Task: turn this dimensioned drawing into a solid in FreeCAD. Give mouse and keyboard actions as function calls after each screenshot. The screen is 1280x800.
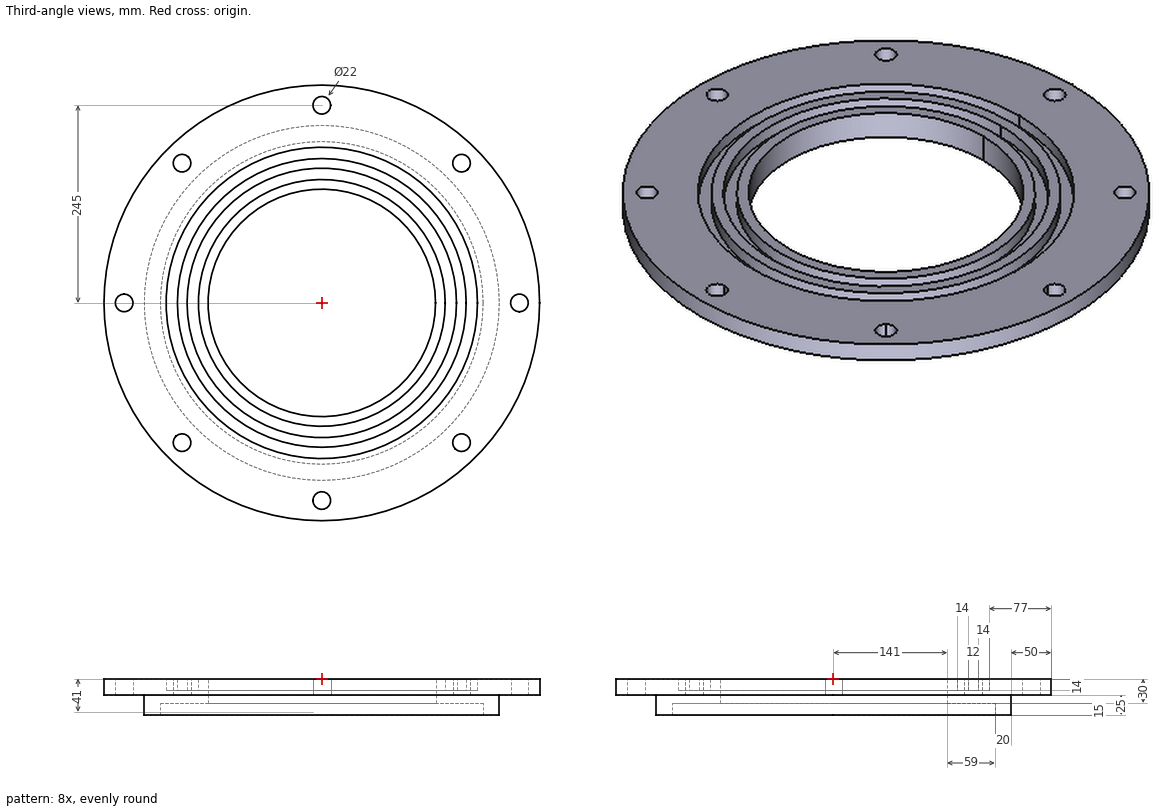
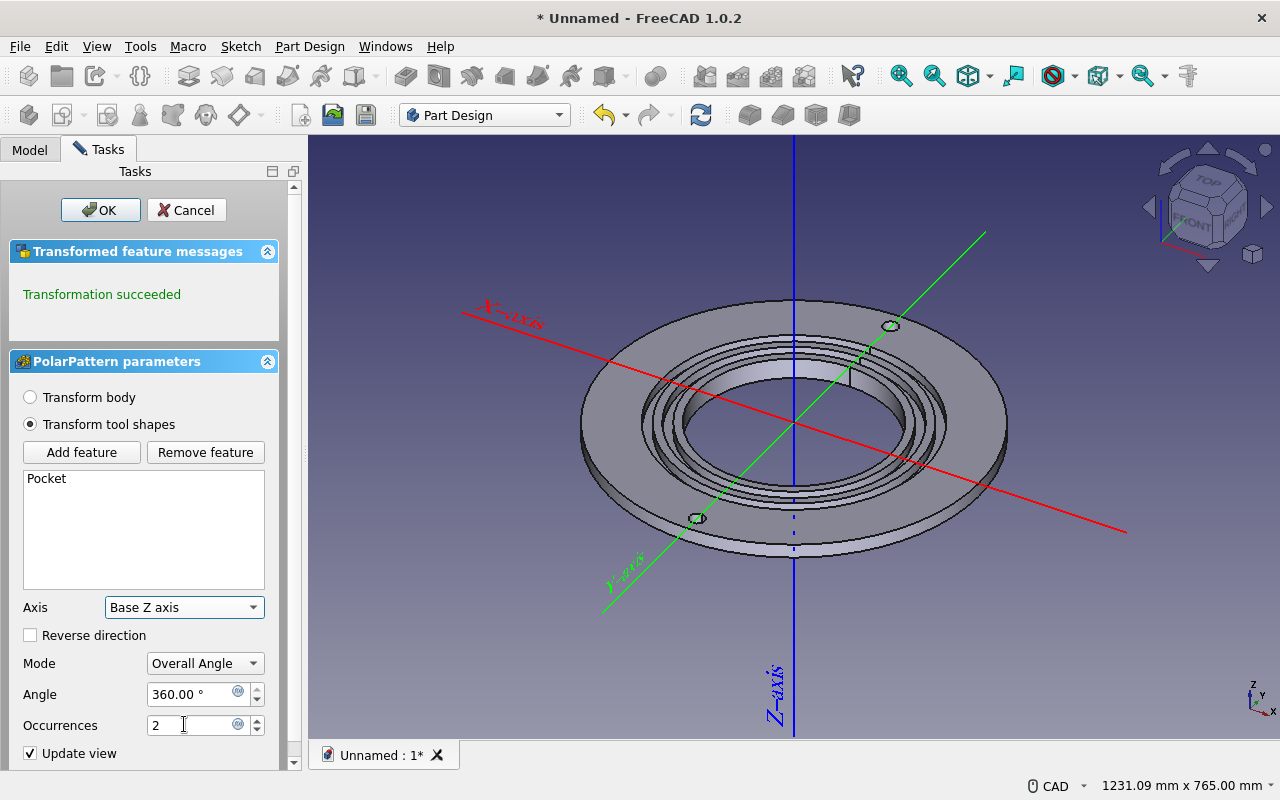
triple_click(199, 726)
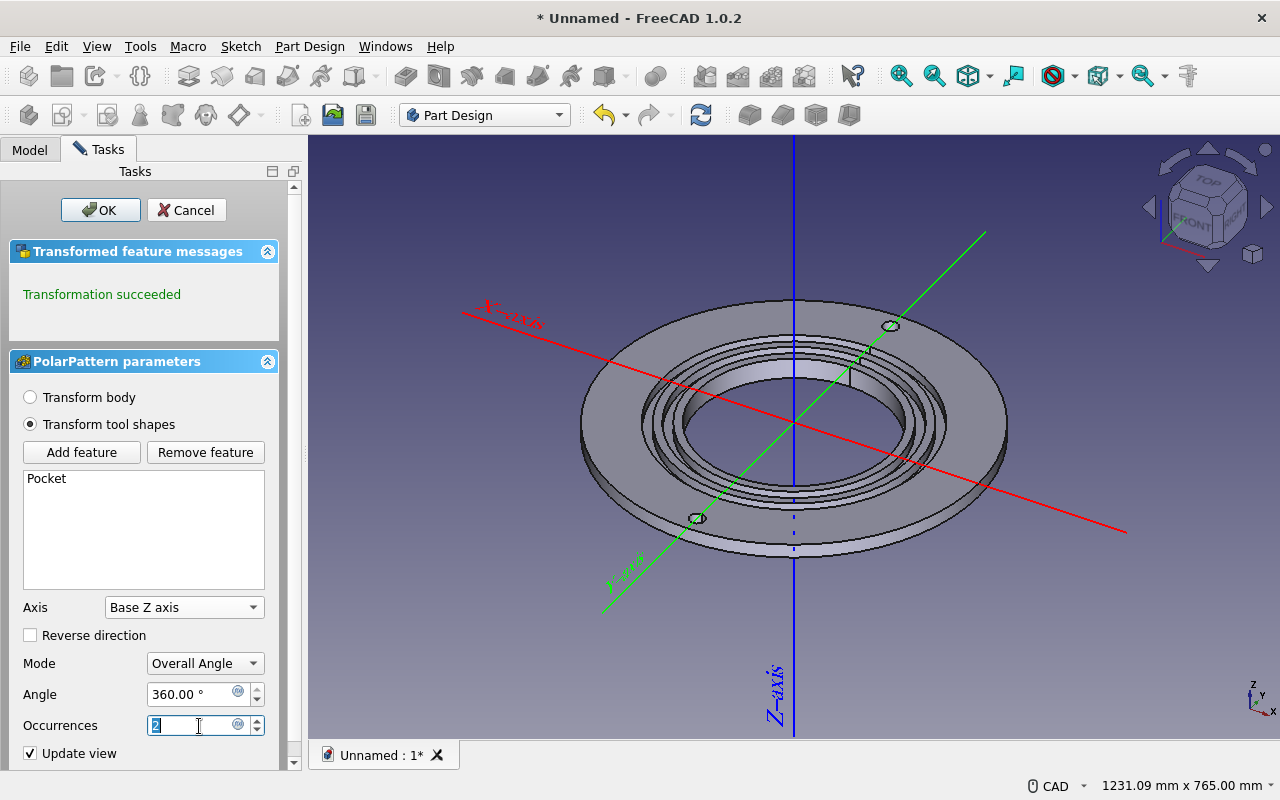
text(8)
key(Tab)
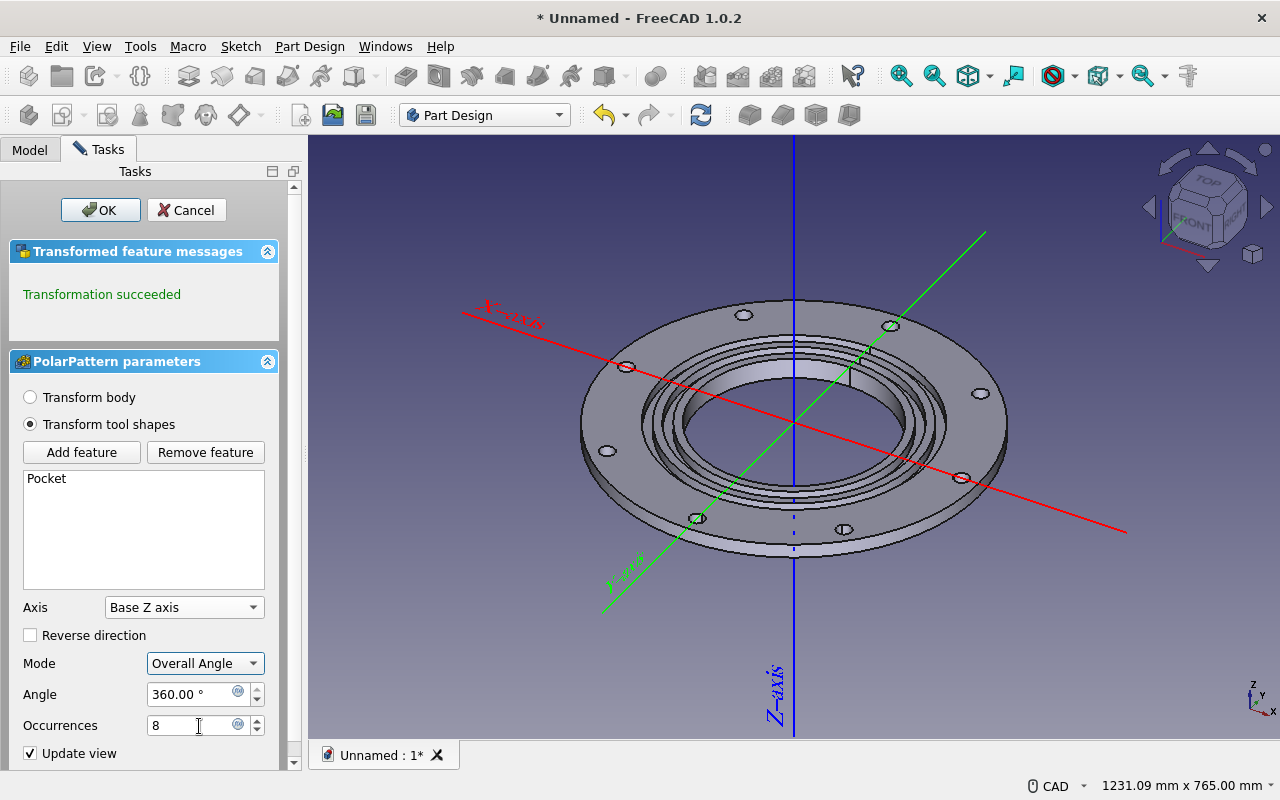
click(101, 210)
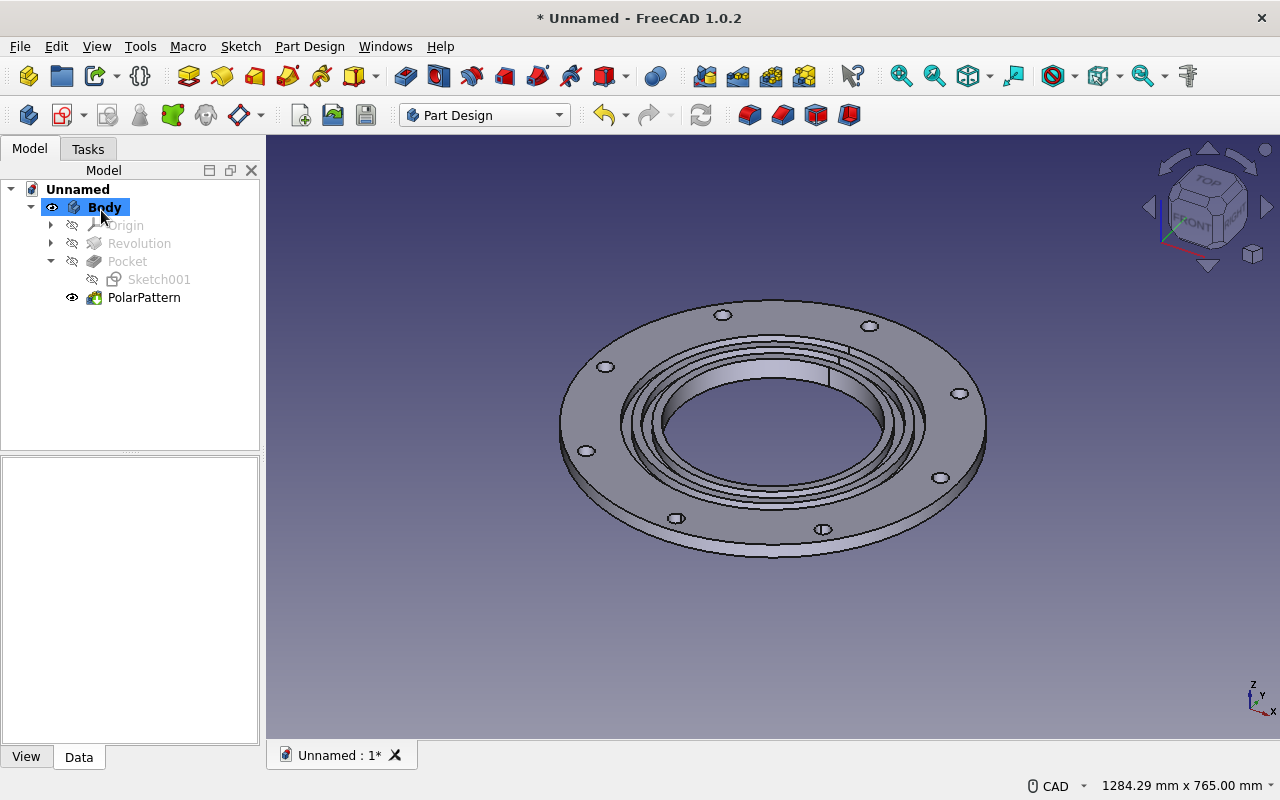
key(0)